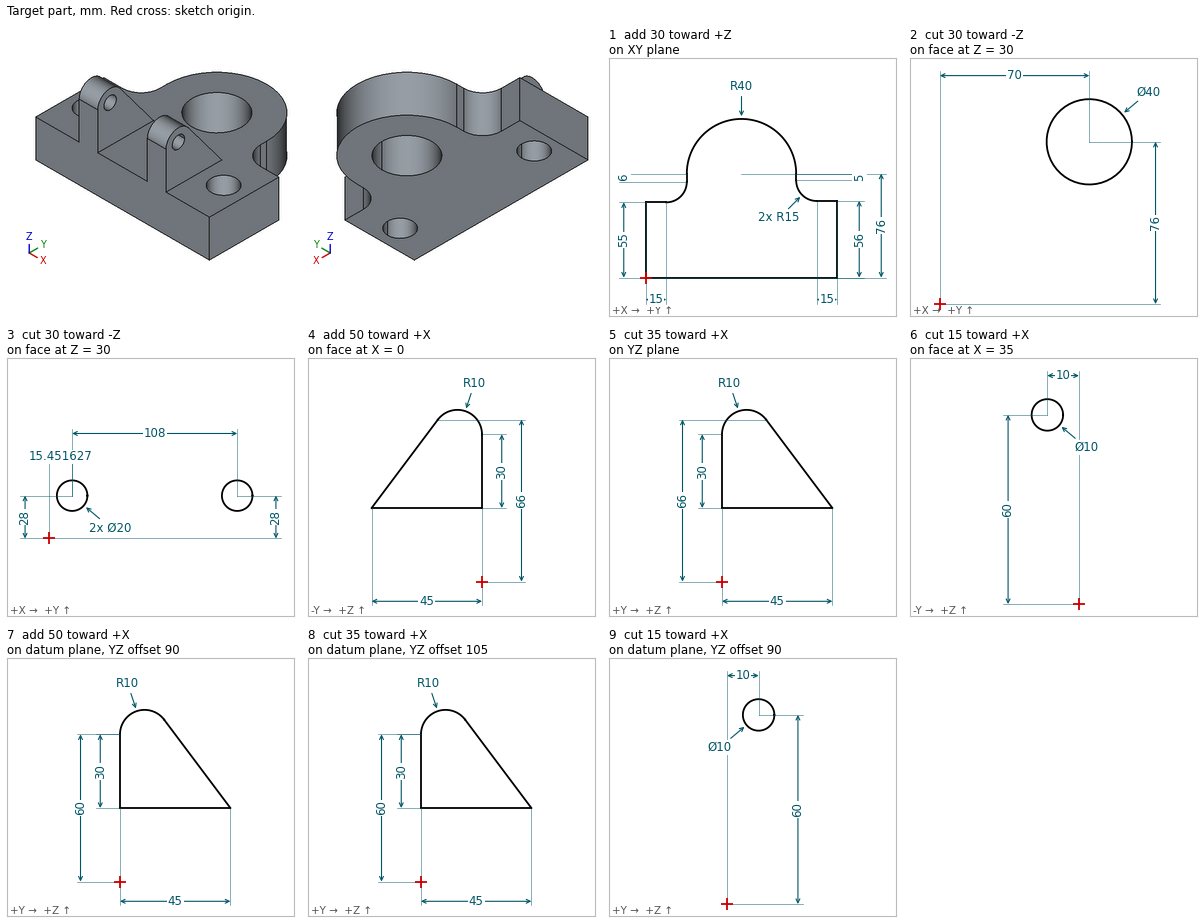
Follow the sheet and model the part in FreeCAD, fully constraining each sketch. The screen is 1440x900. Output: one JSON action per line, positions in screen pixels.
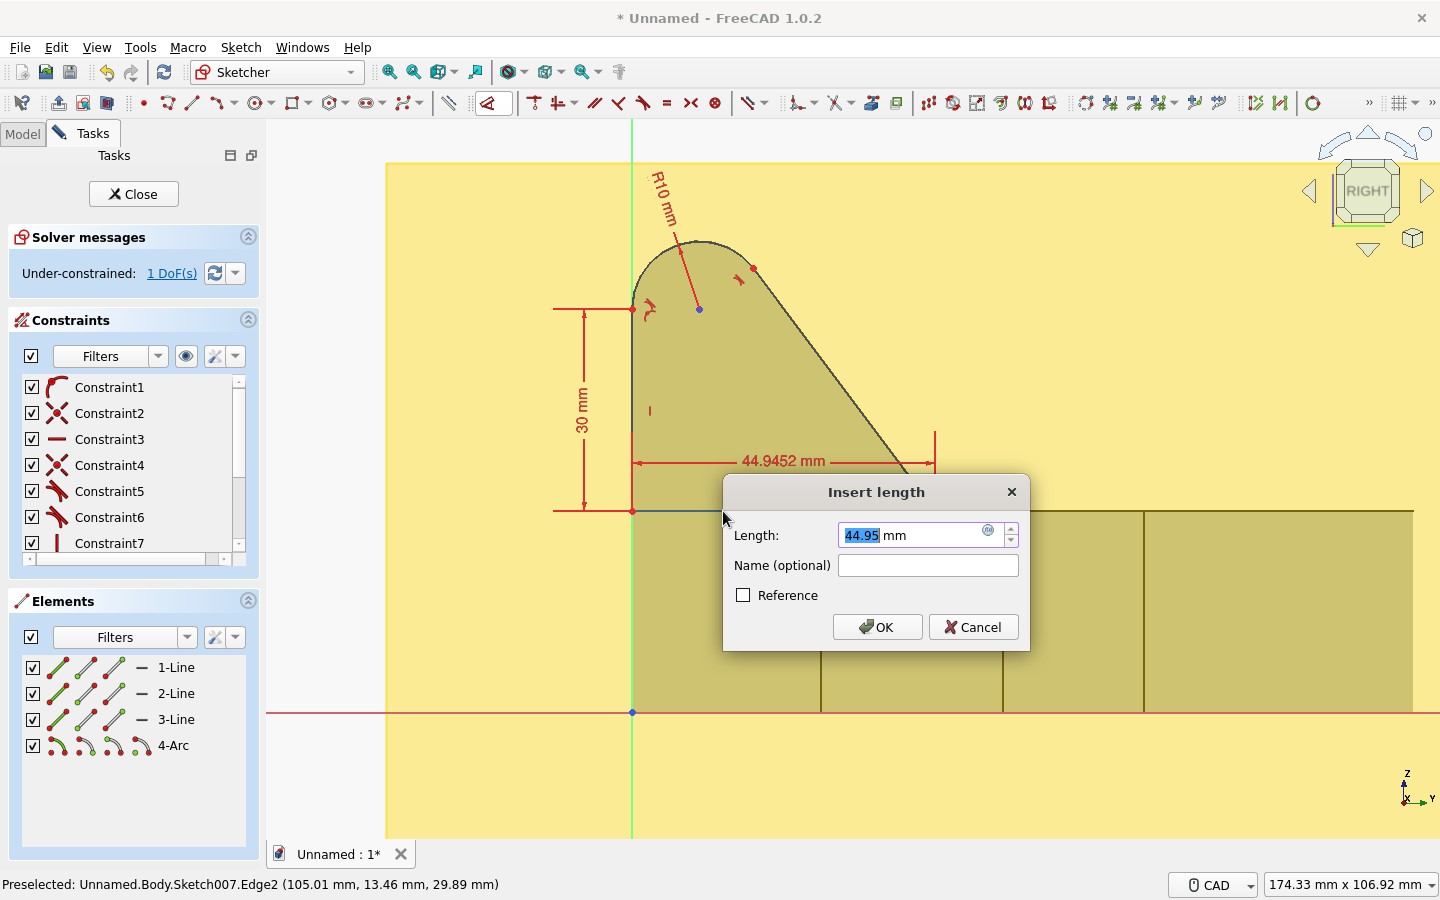
{"action": "type", "text": "45"}
{"action": "key", "text": "Return"}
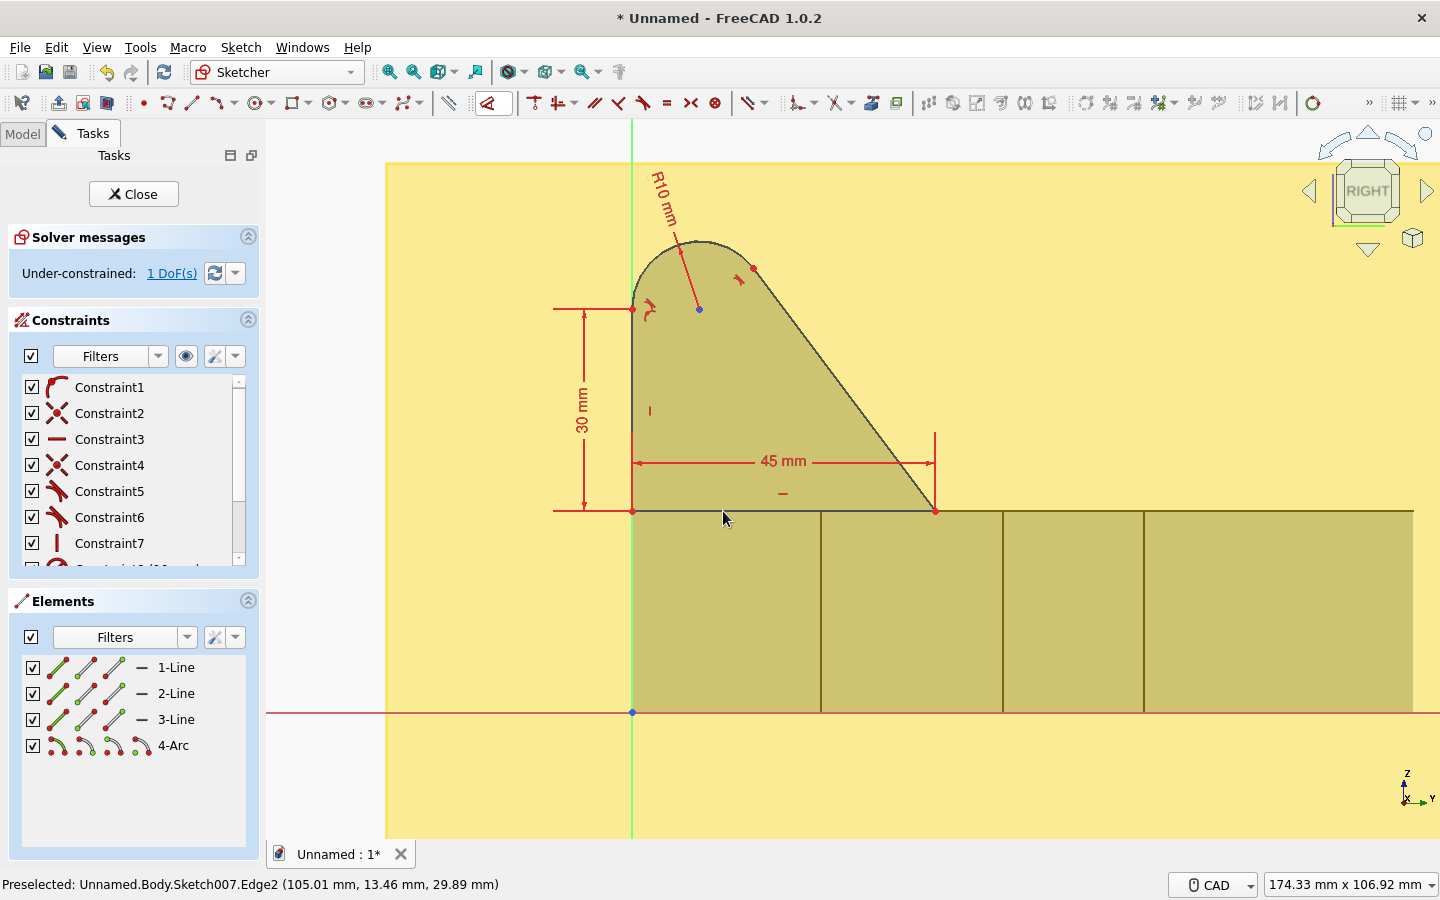
{"action": "left_click", "coordinate": [632, 309]}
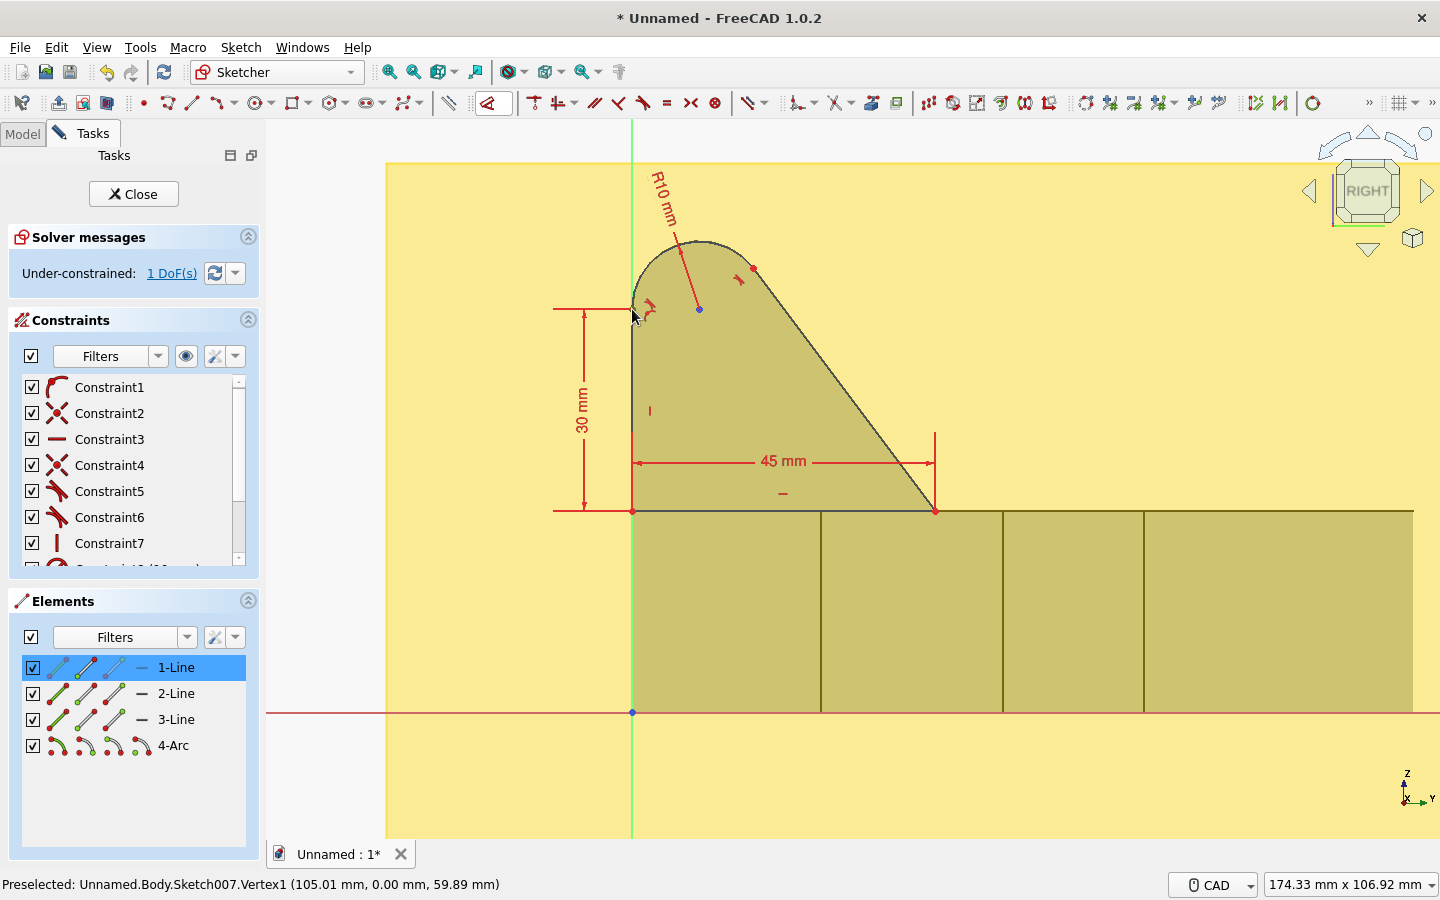
{"action": "key", "text": "i"}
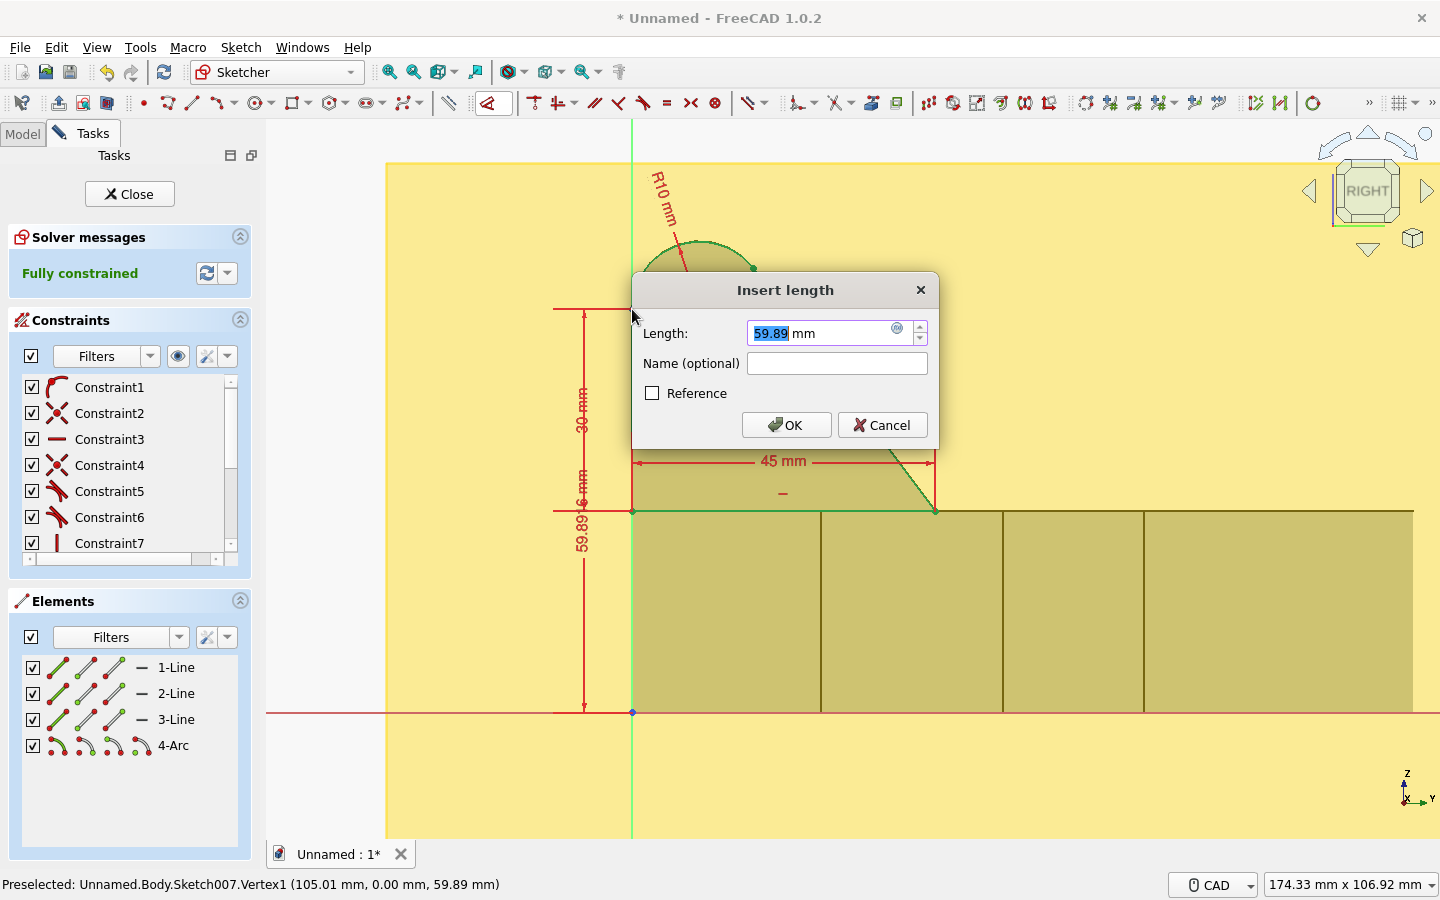
{"action": "type", "text": "60"}
{"action": "key", "text": "Return"}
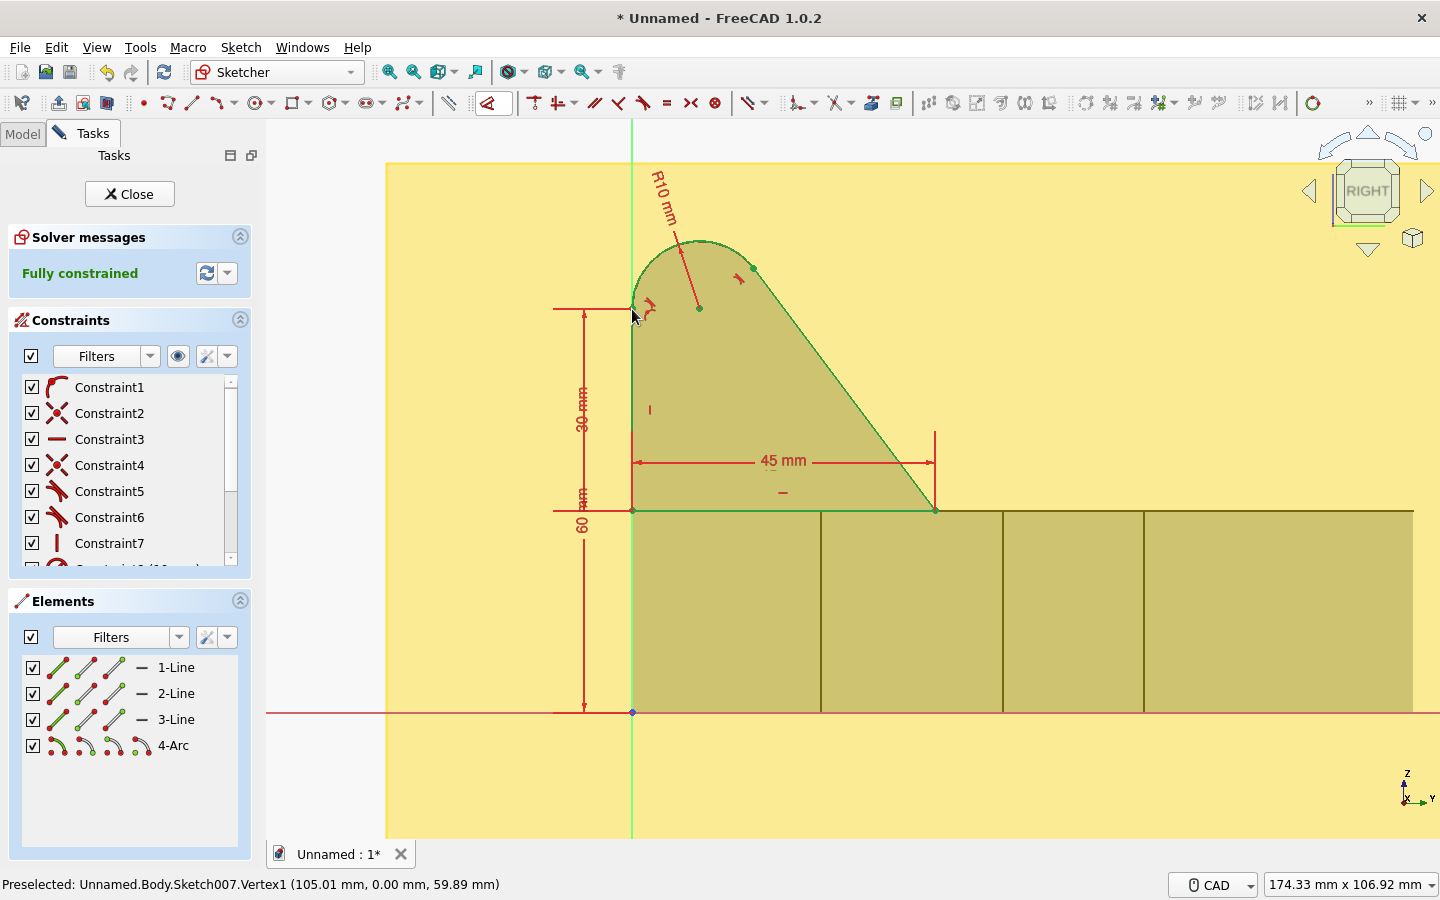
{"action": "left_click", "coordinate": [130, 194]}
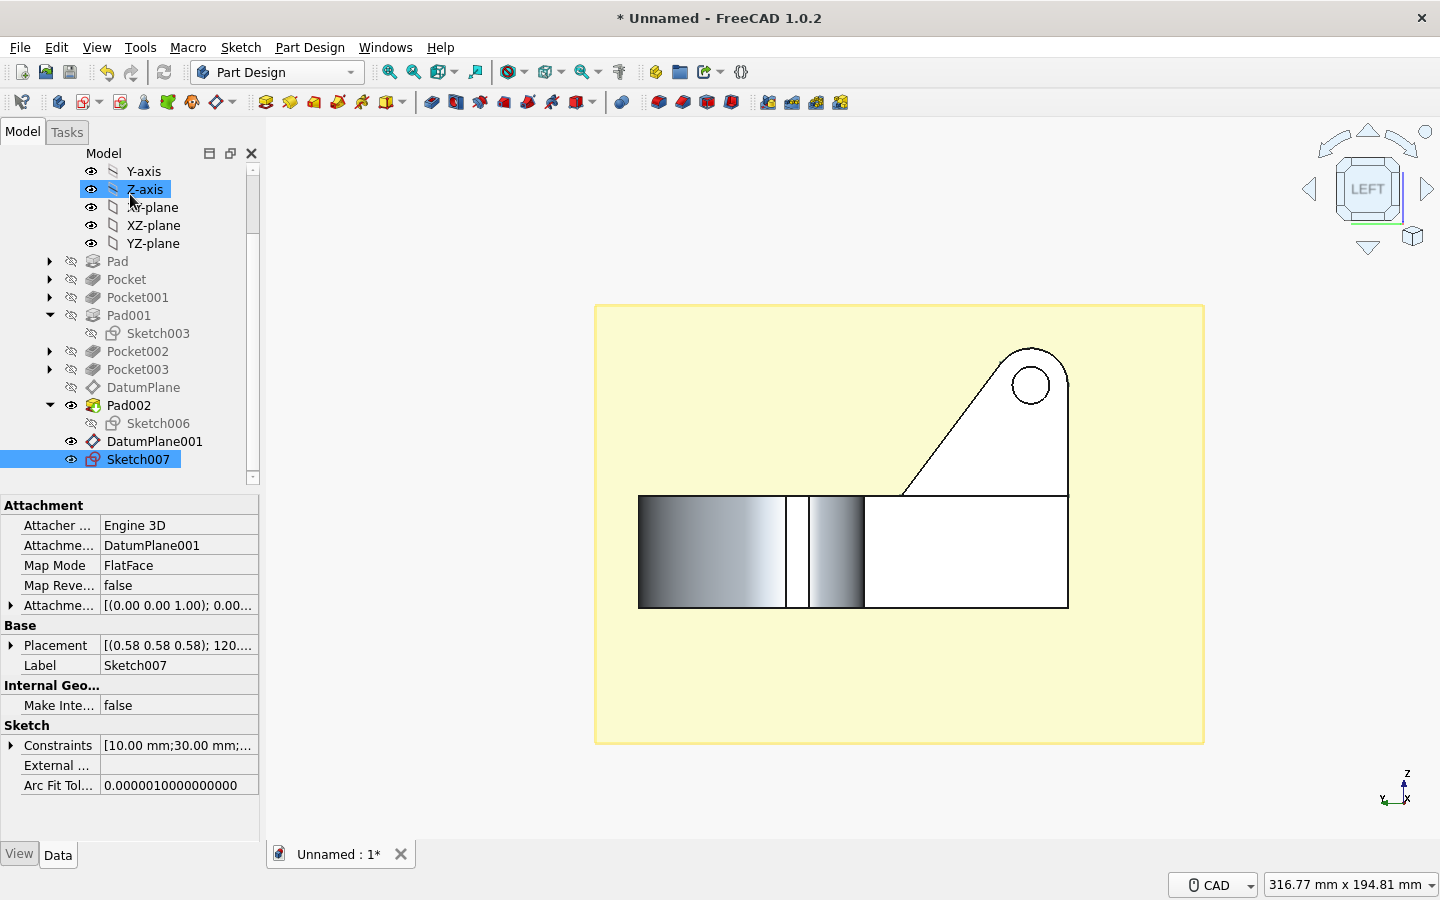
{"action": "left_click", "coordinate": [432, 102]}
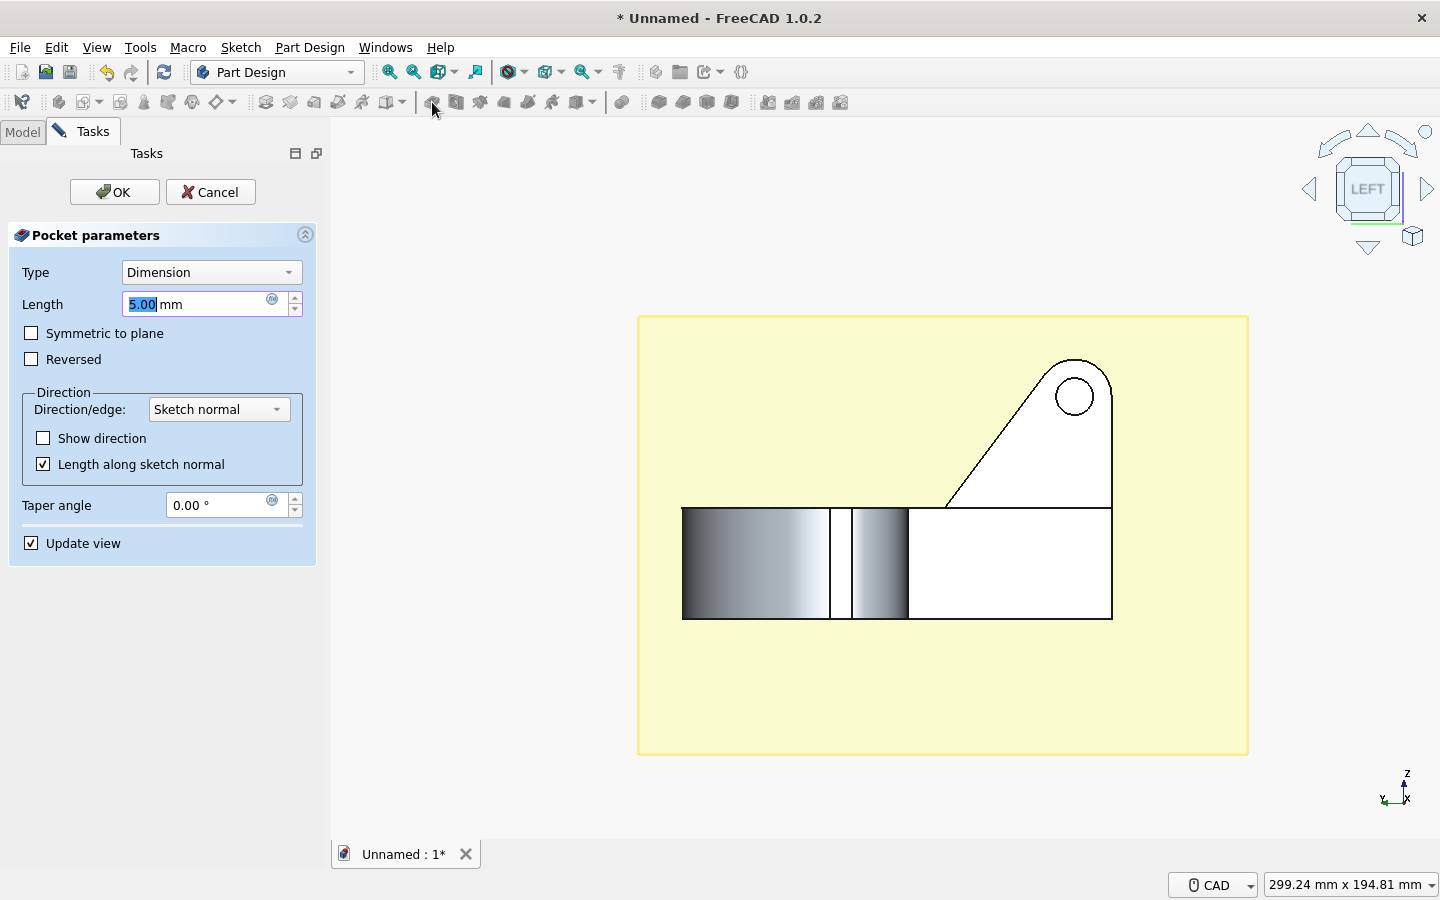
{"action": "type", "text": "35"}
{"action": "key", "text": "Tab"}